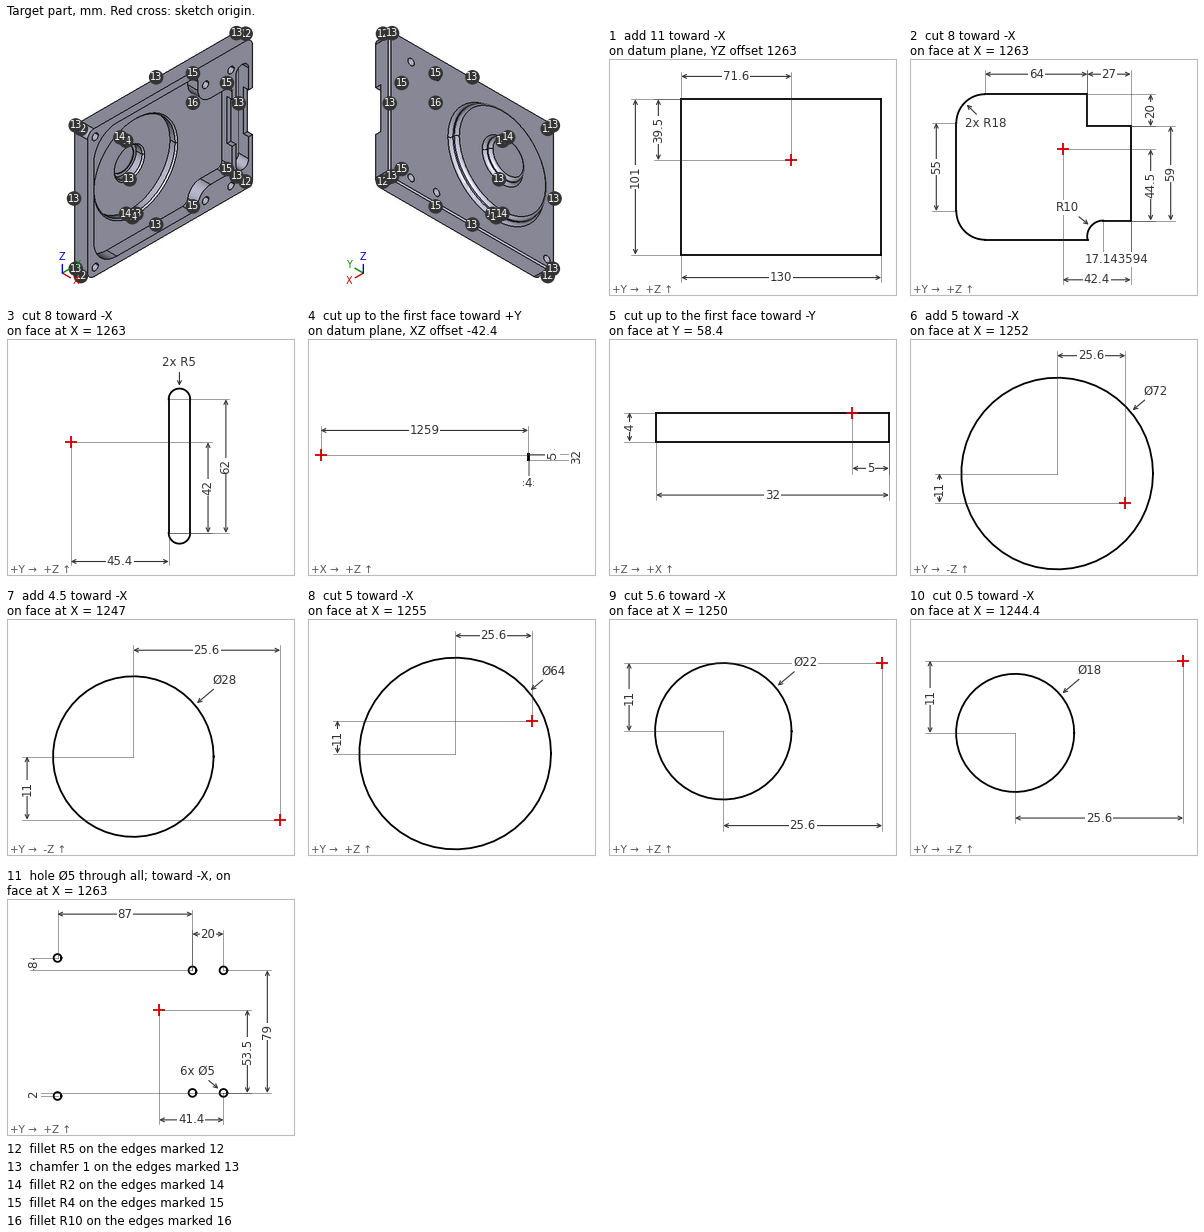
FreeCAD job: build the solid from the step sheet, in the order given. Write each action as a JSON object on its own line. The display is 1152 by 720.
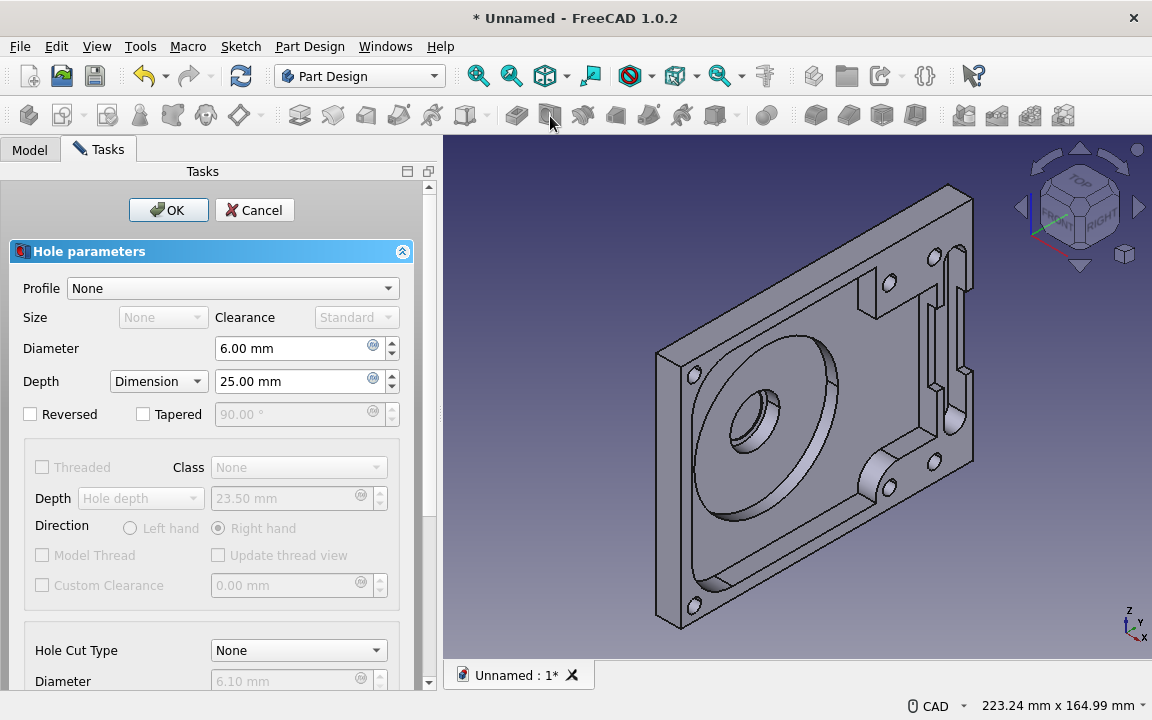
{"action": "triple_click", "coordinate": [300, 348]}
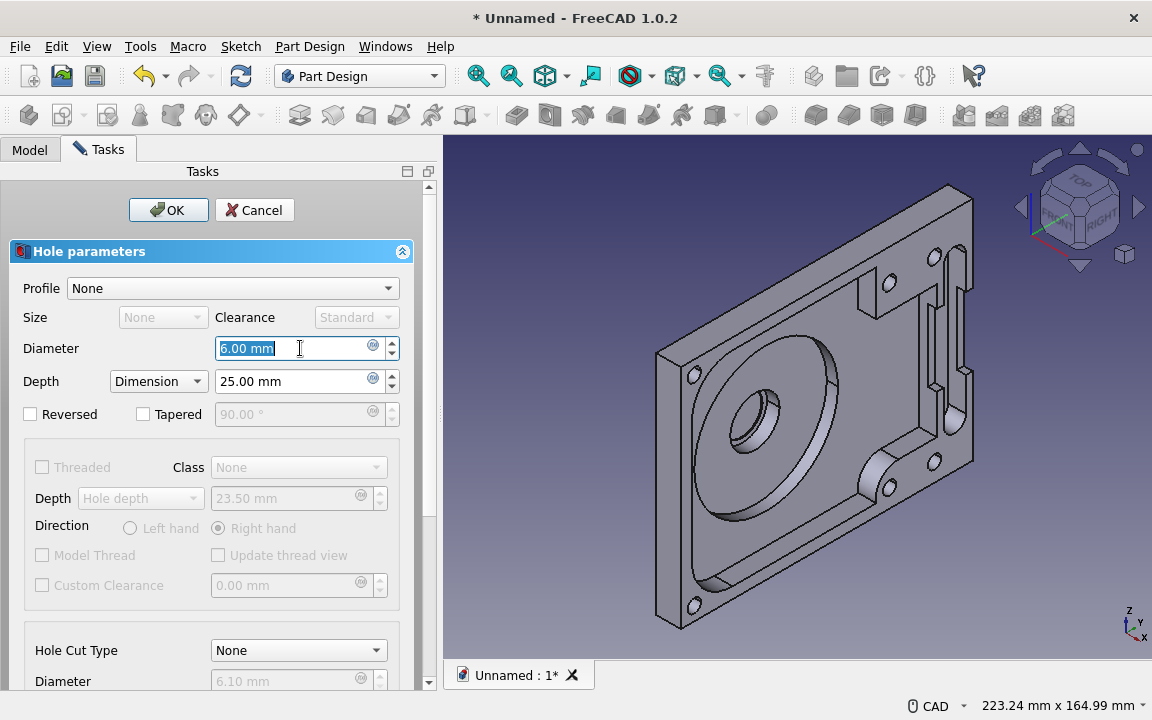
{"action": "type", "text": "5"}
{"action": "key", "text": "Tab"}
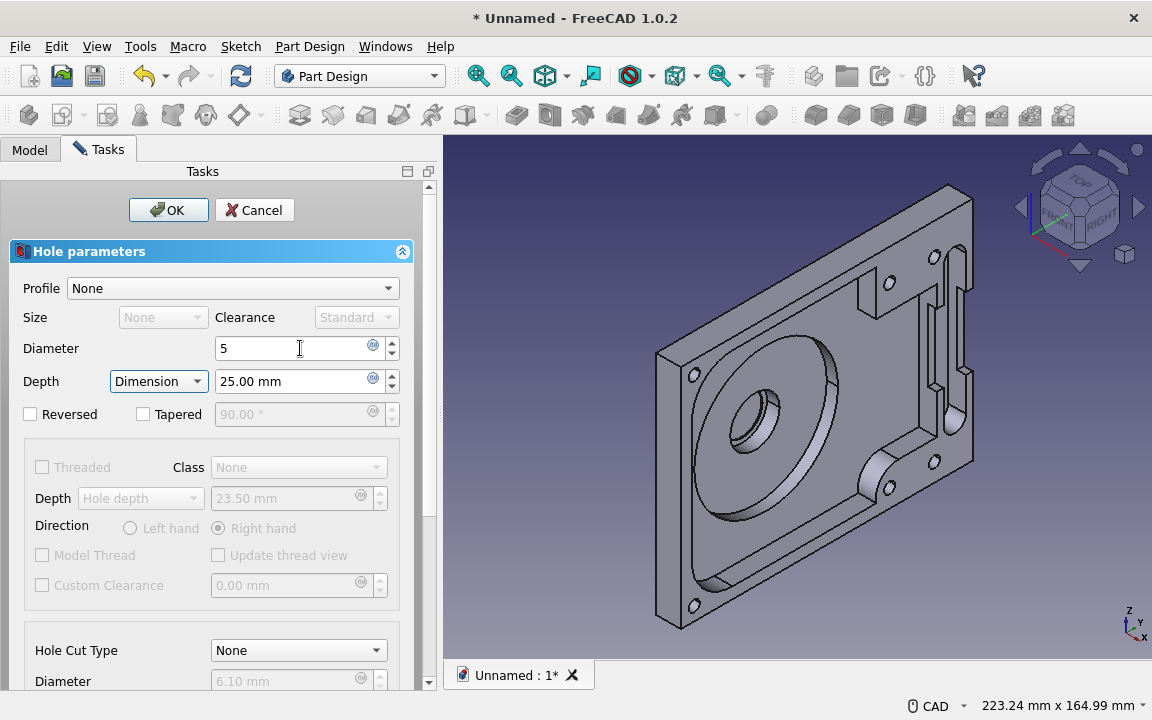
{"action": "left_click", "coordinate": [160, 382]}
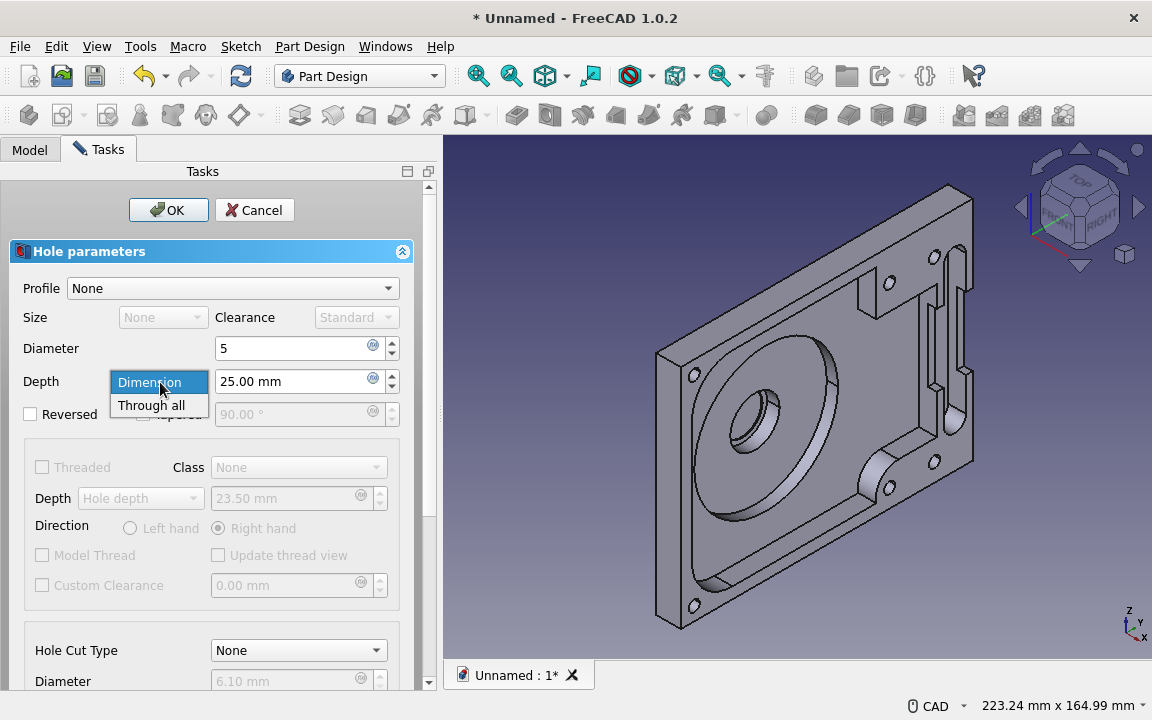
{"action": "left_click", "coordinate": [158, 406]}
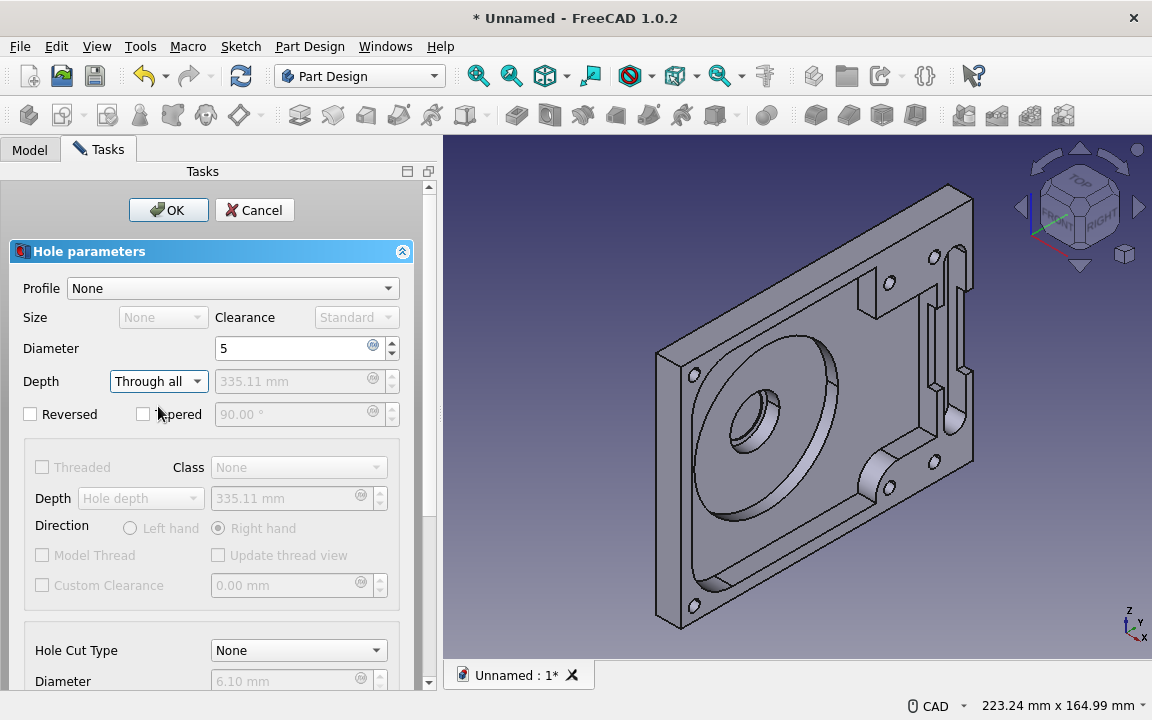
{"action": "left_click", "coordinate": [169, 210]}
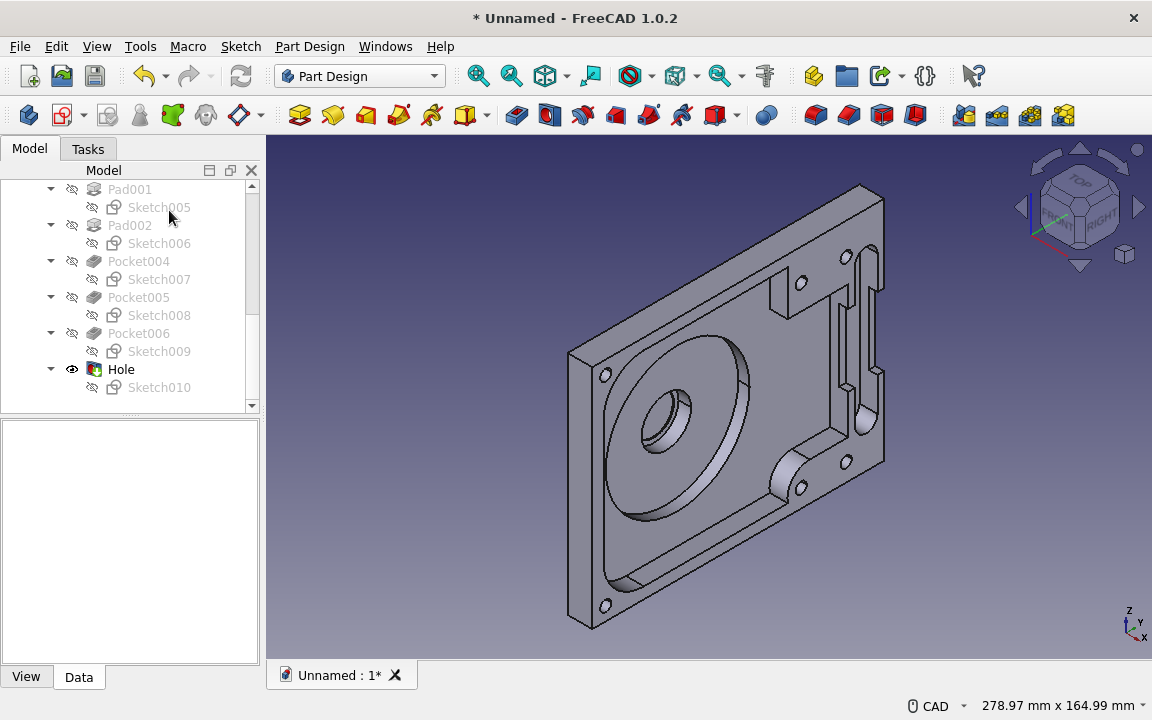
{"action": "left_click", "coordinate": [580, 359]}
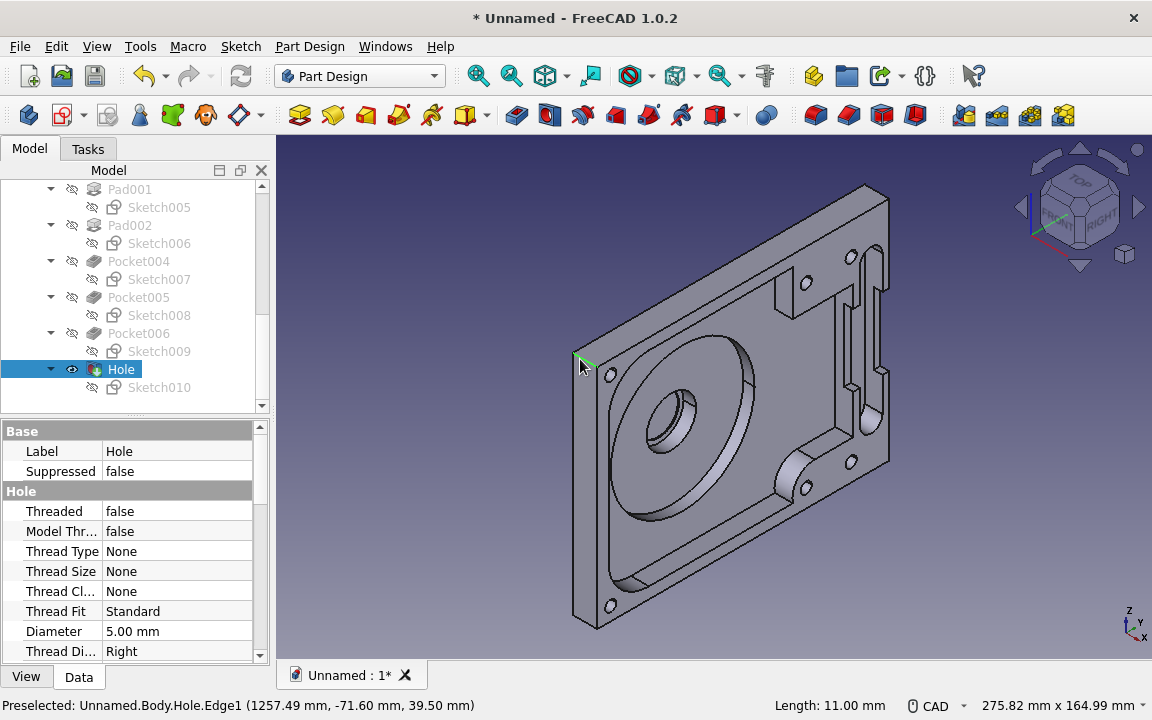
{"action": "key", "text": "2"}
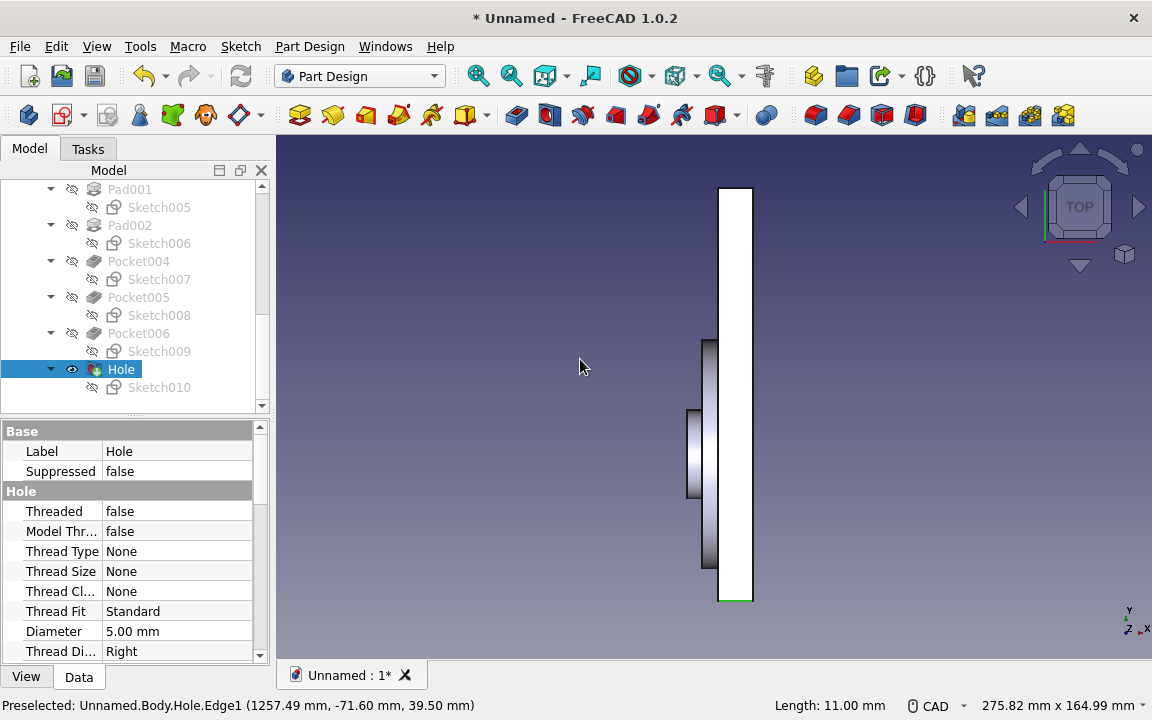
{"action": "left_click", "coordinate": [735, 187], "text": "ctrl"}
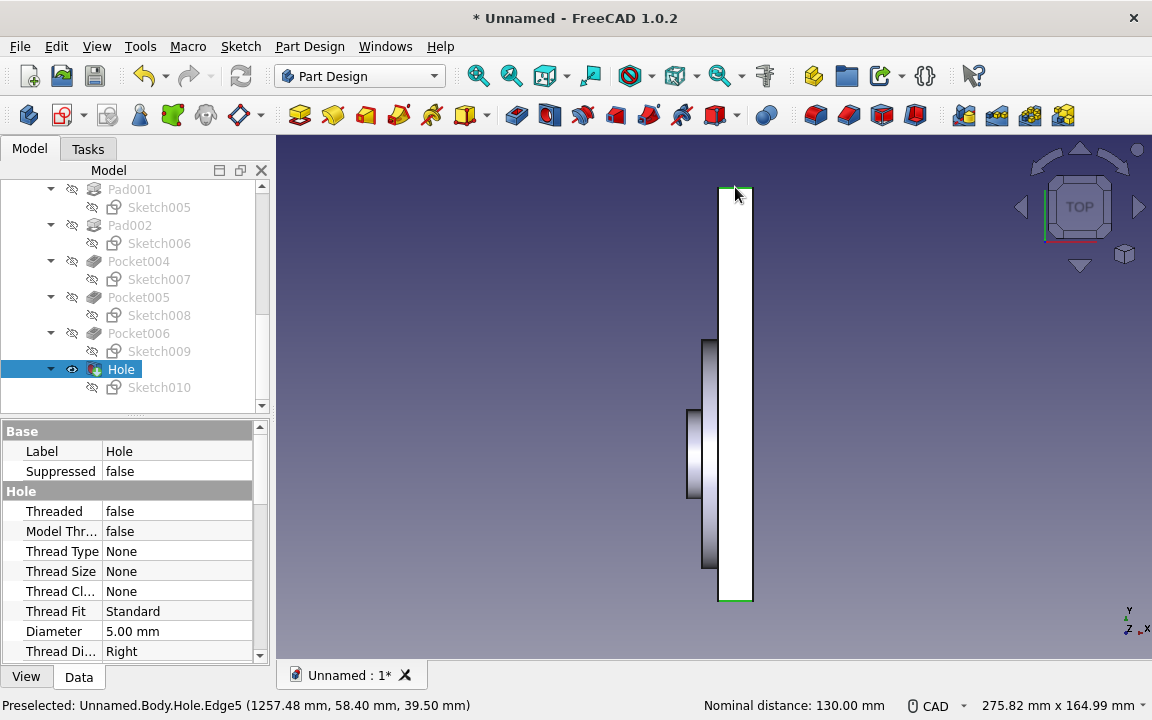
{"action": "key", "text": "0"}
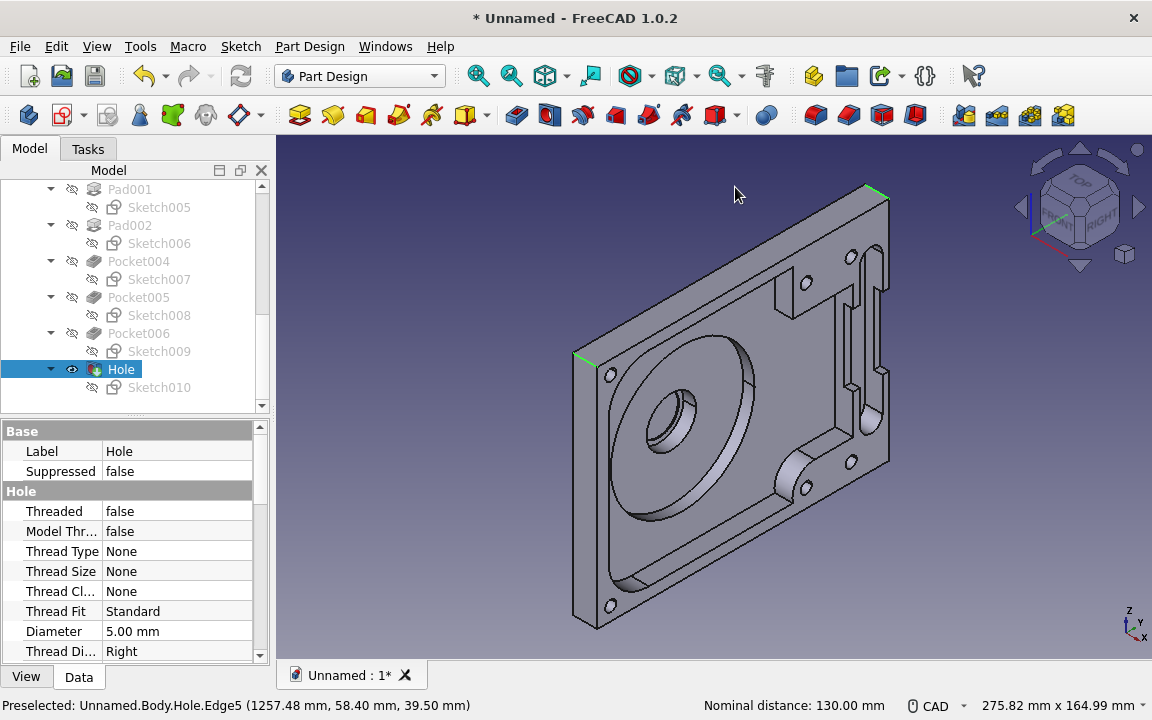
{"action": "key", "text": "1"}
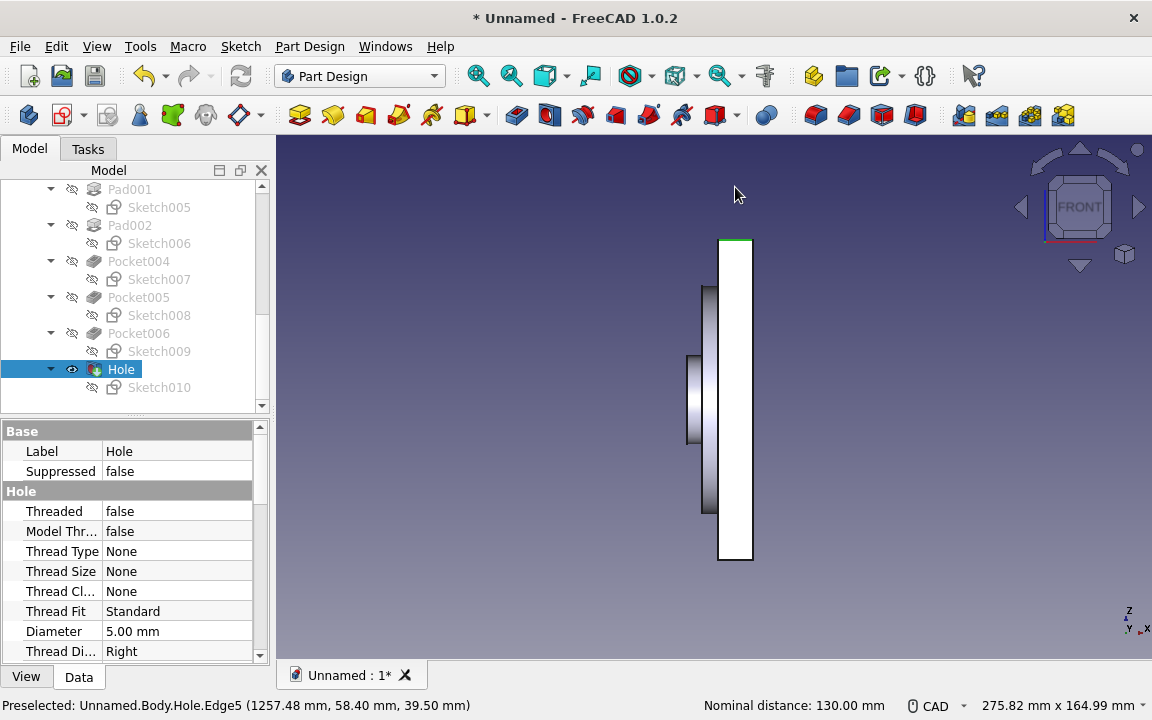
{"action": "left_click", "coordinate": [735, 559], "text": "ctrl"}